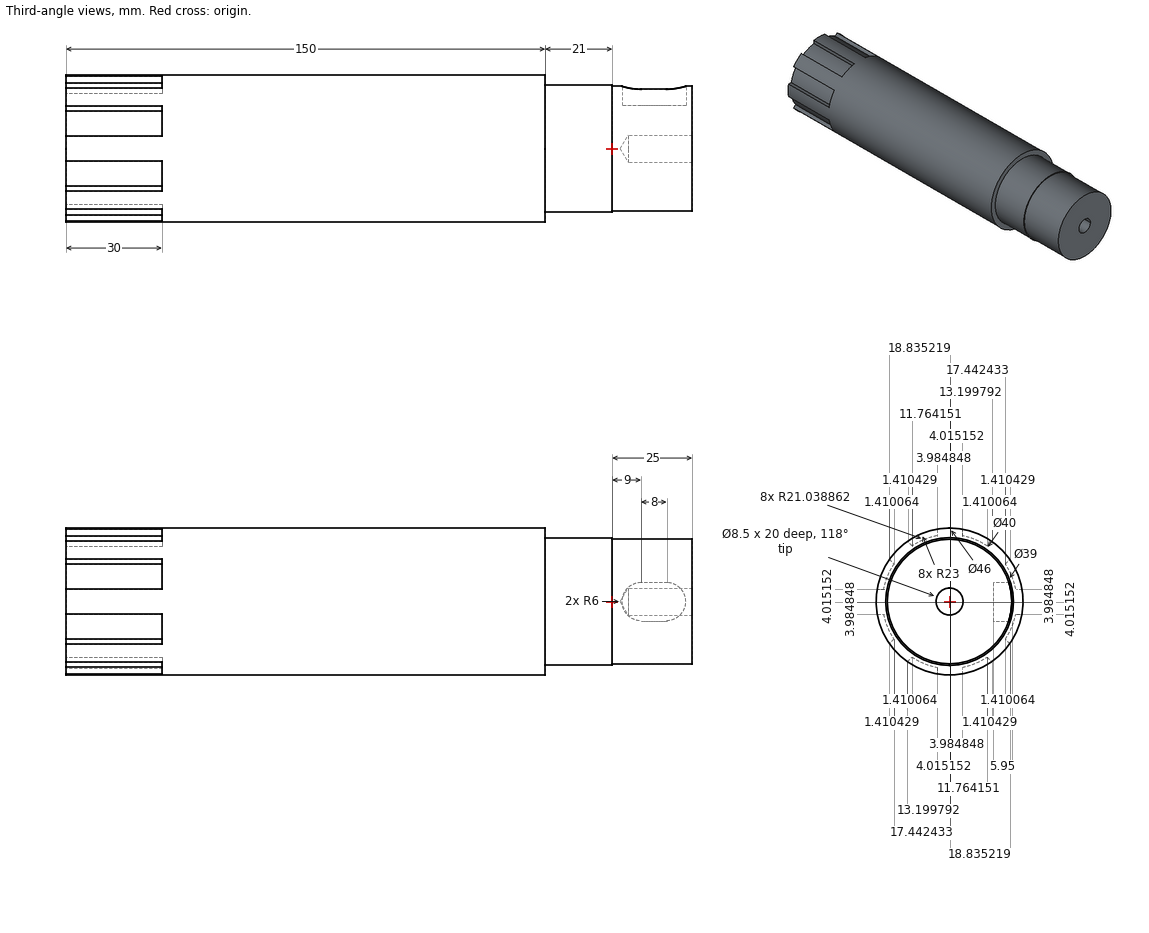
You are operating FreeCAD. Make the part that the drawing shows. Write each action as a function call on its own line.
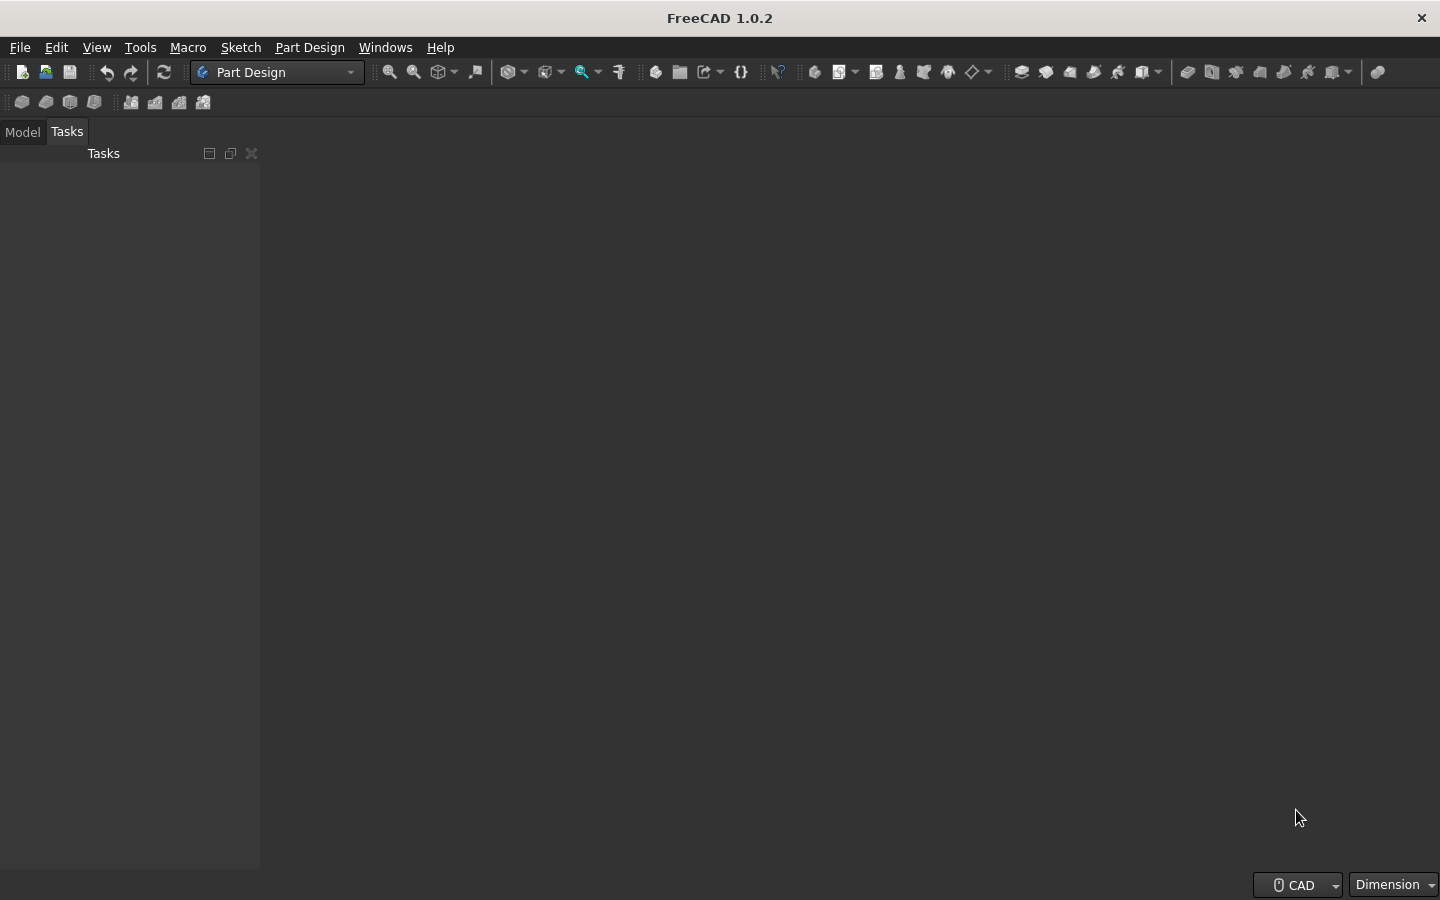
click(22, 72)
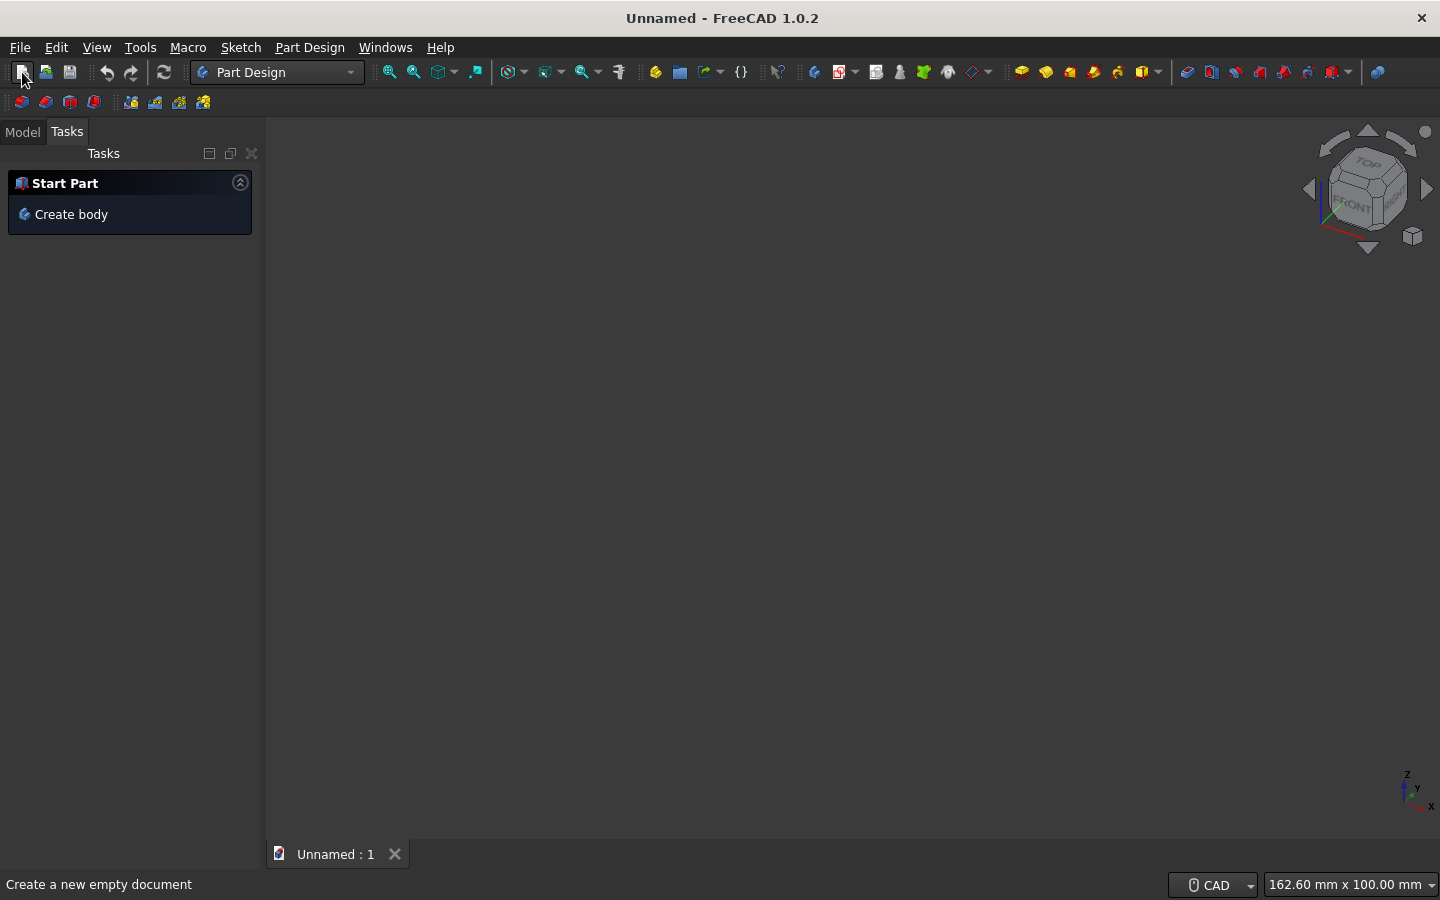
click(840, 72)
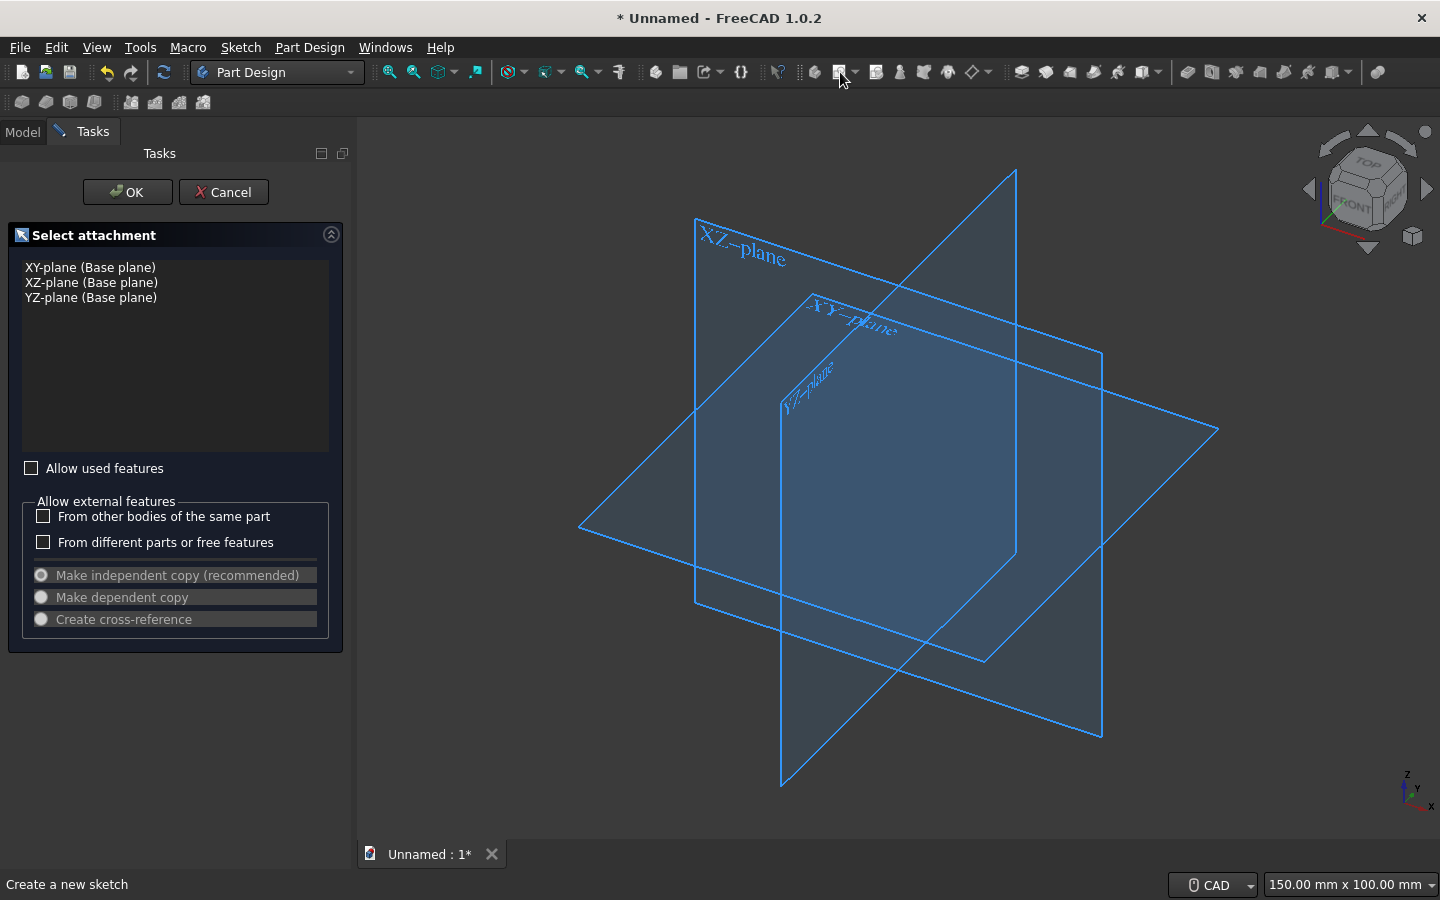
click(82, 298)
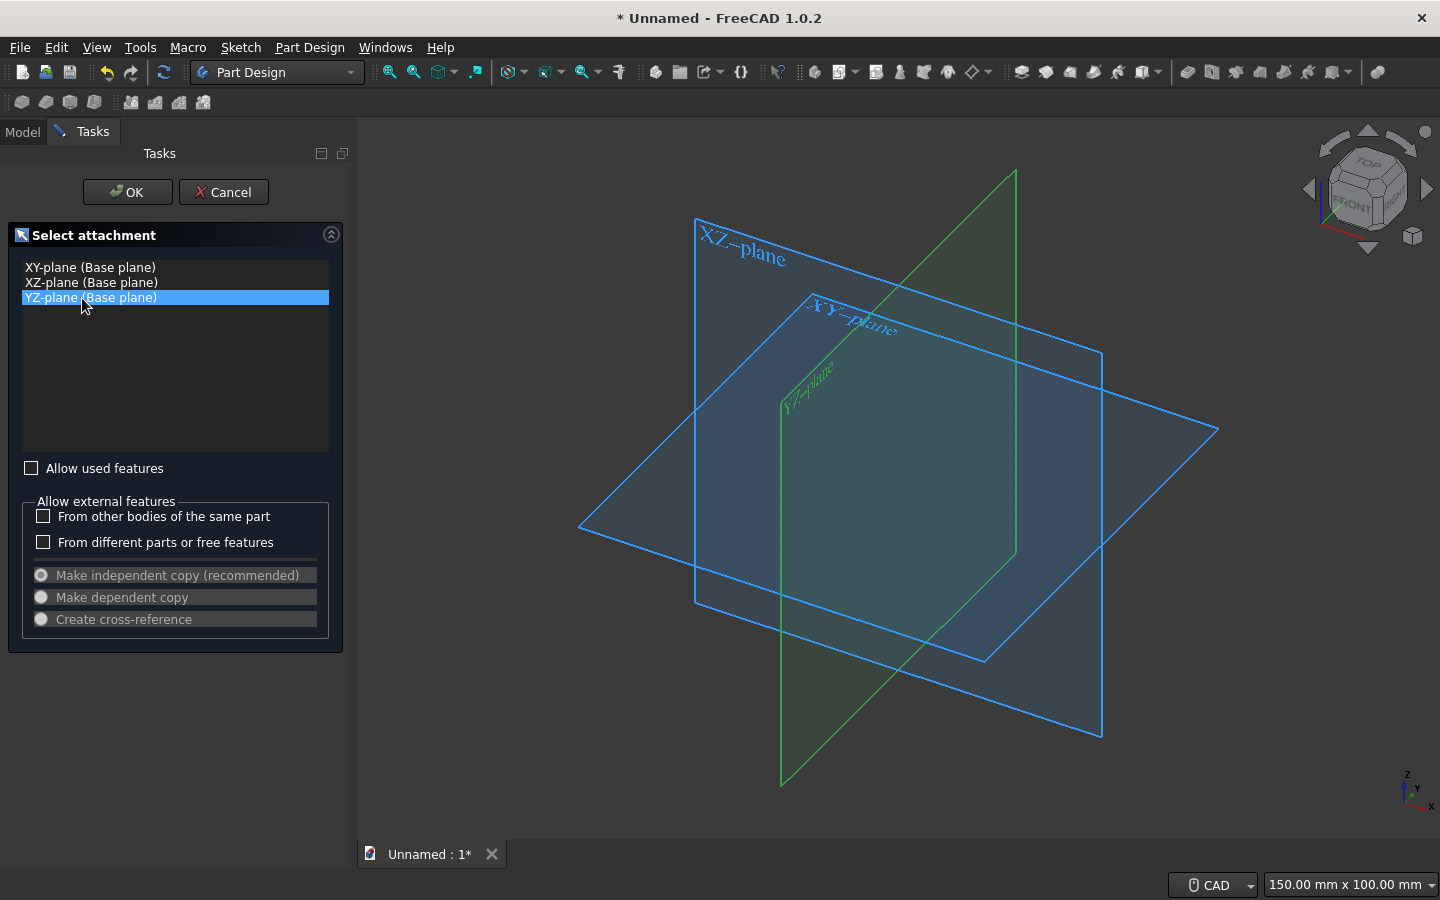
click(128, 192)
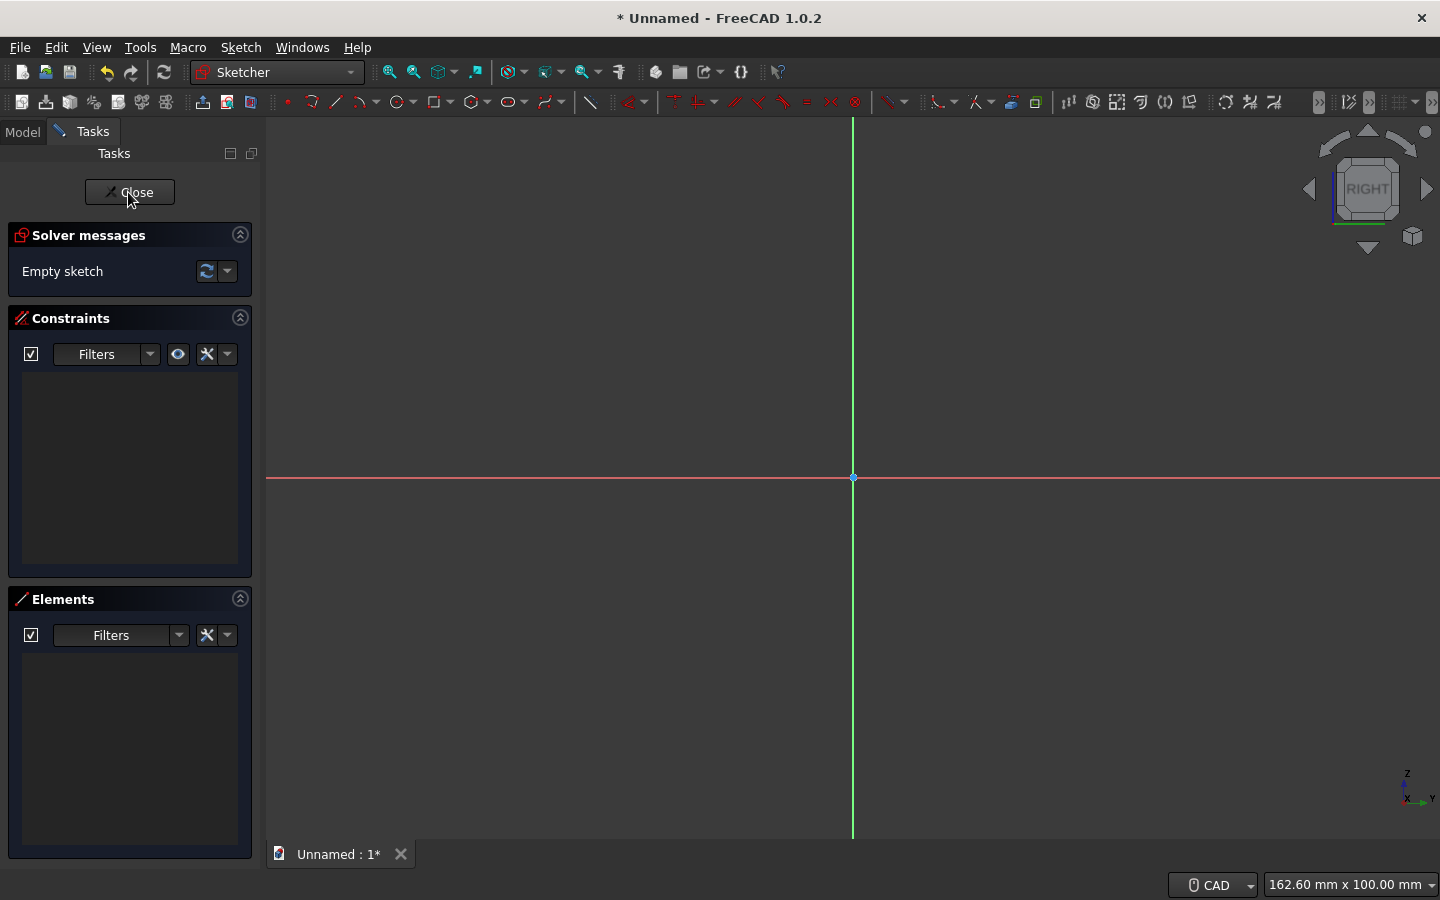
scroll(936, 478, up, 3)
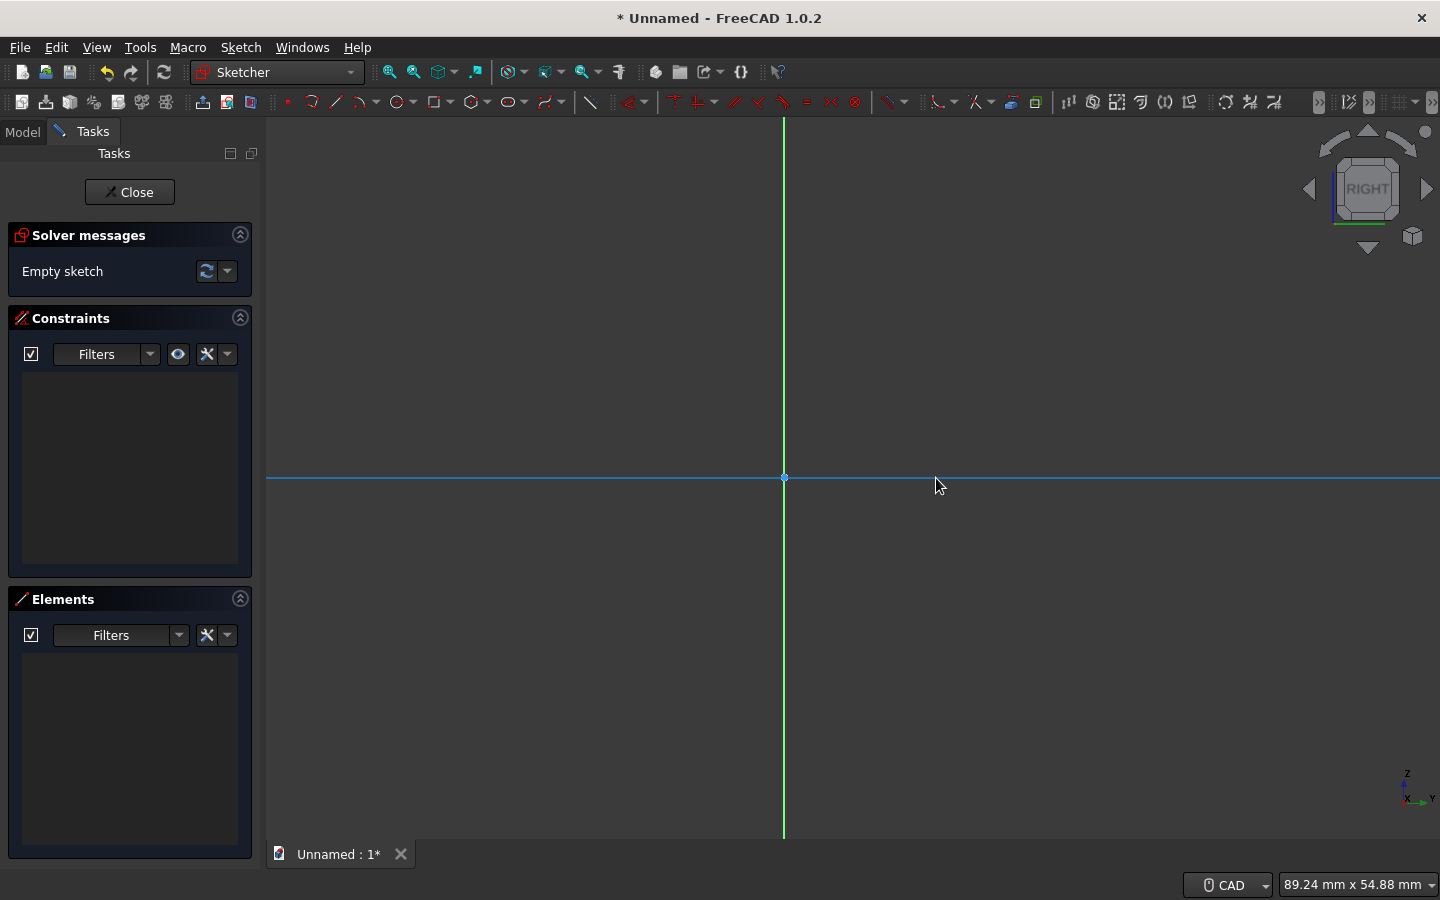
click(398, 102)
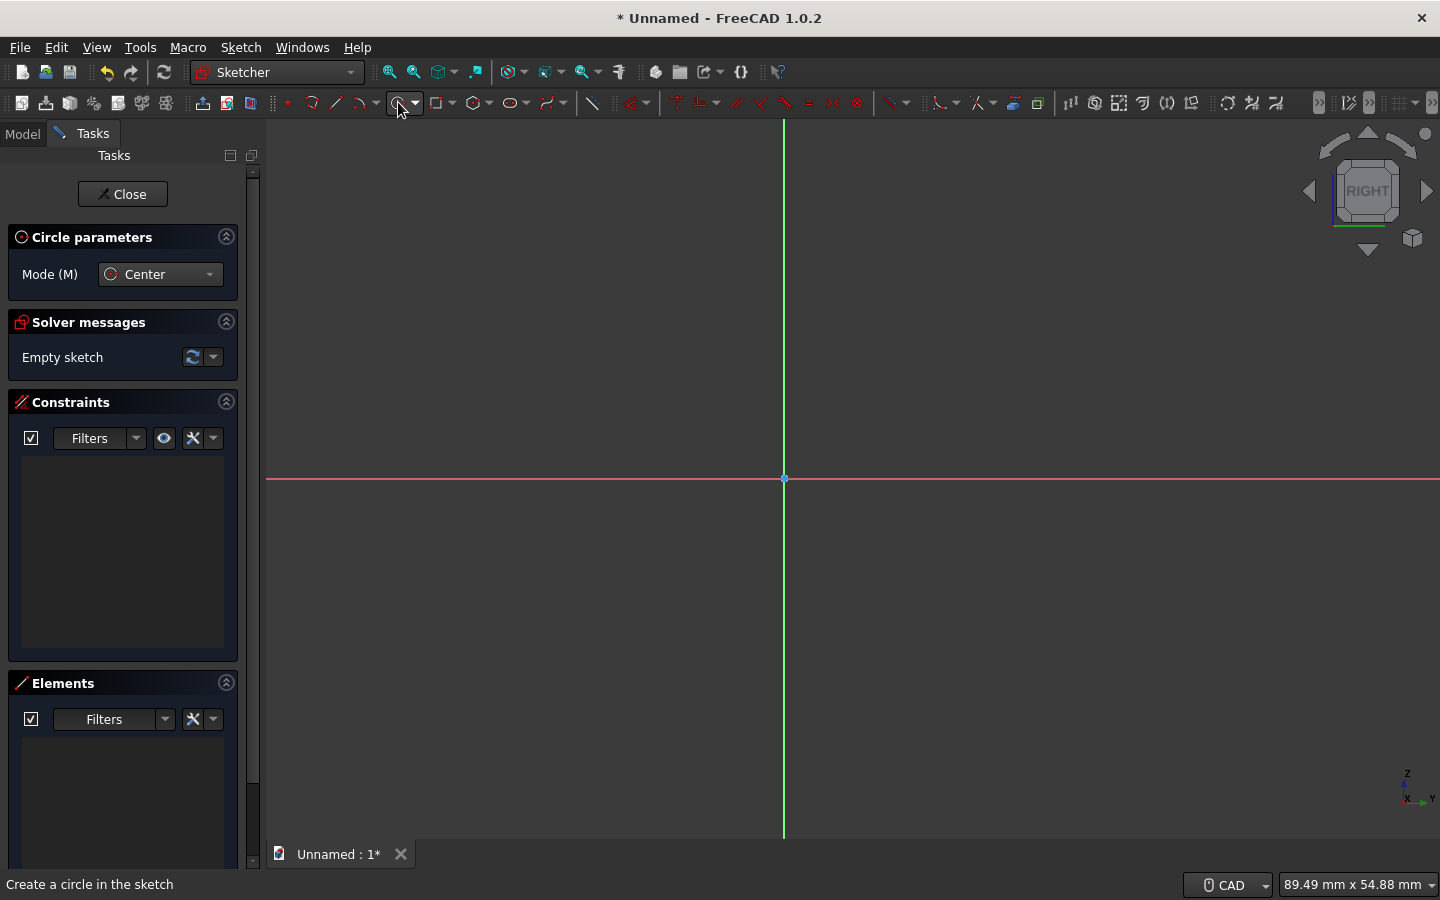
click(784, 479)
click(965, 298)
key(Escape)